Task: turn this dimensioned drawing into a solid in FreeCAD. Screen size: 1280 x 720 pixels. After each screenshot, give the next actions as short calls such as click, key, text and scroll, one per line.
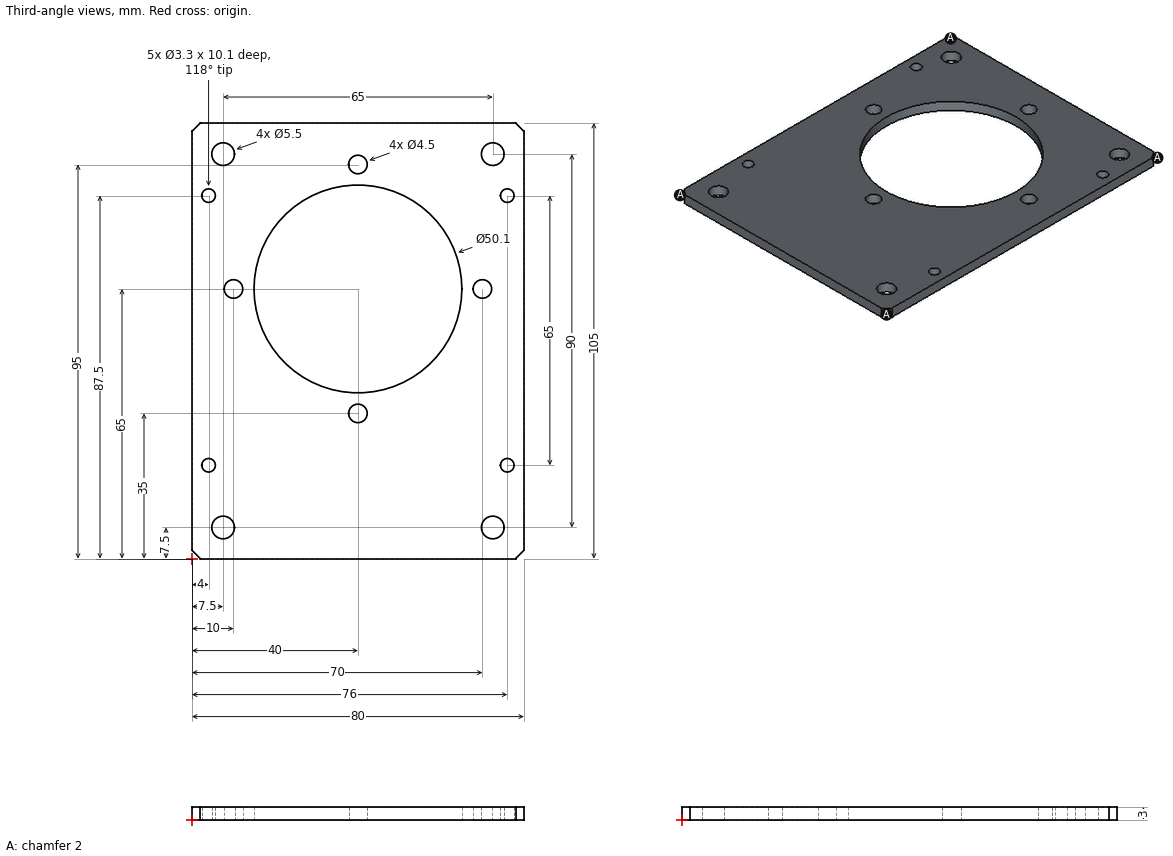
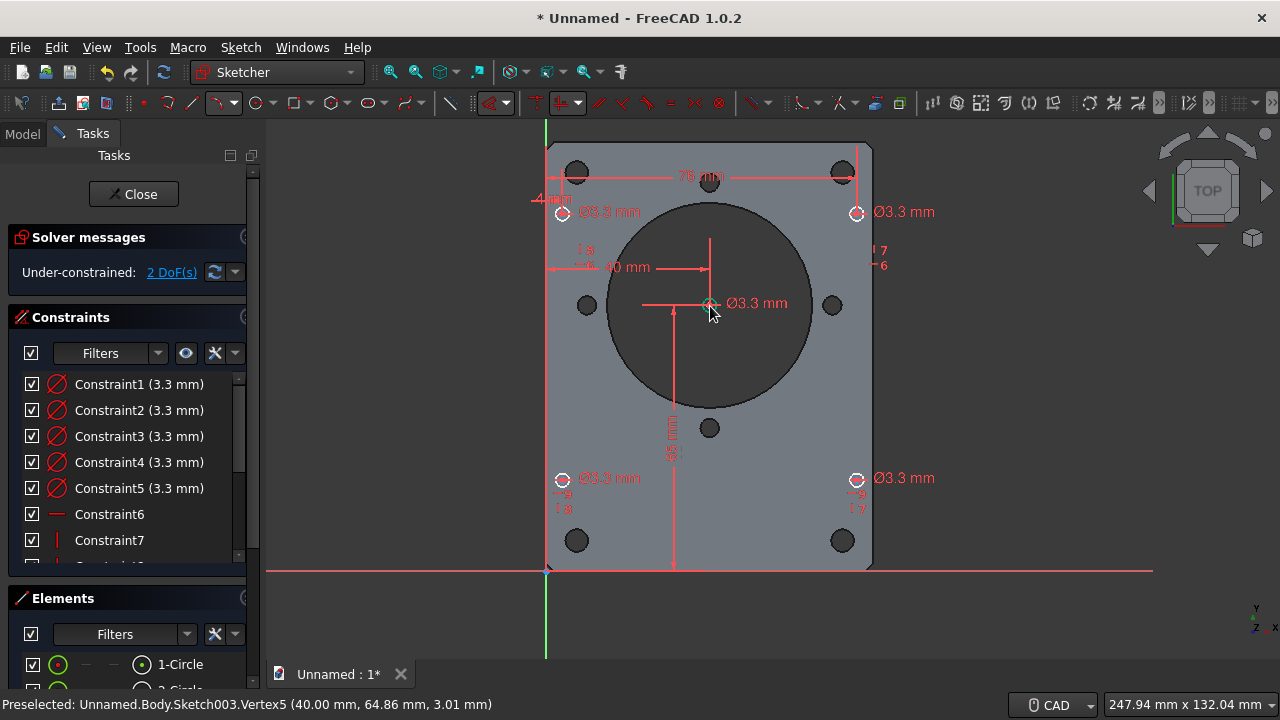
click(857, 214)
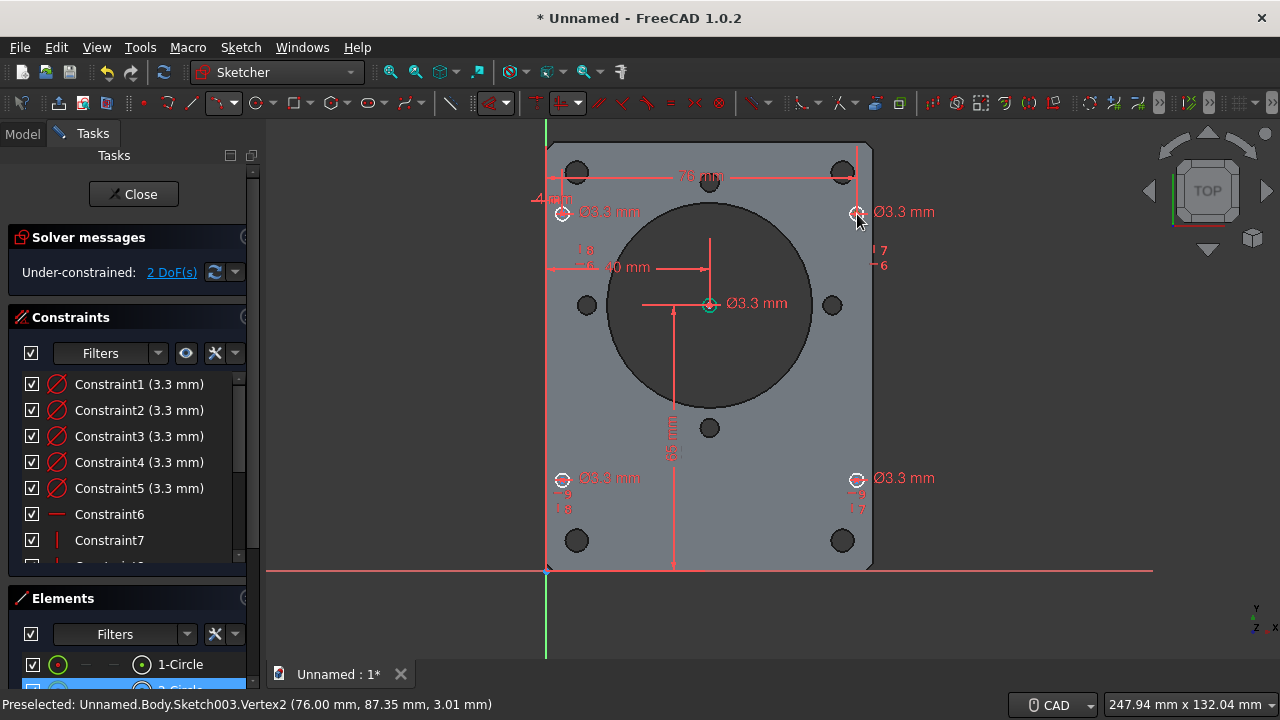
click(857, 480)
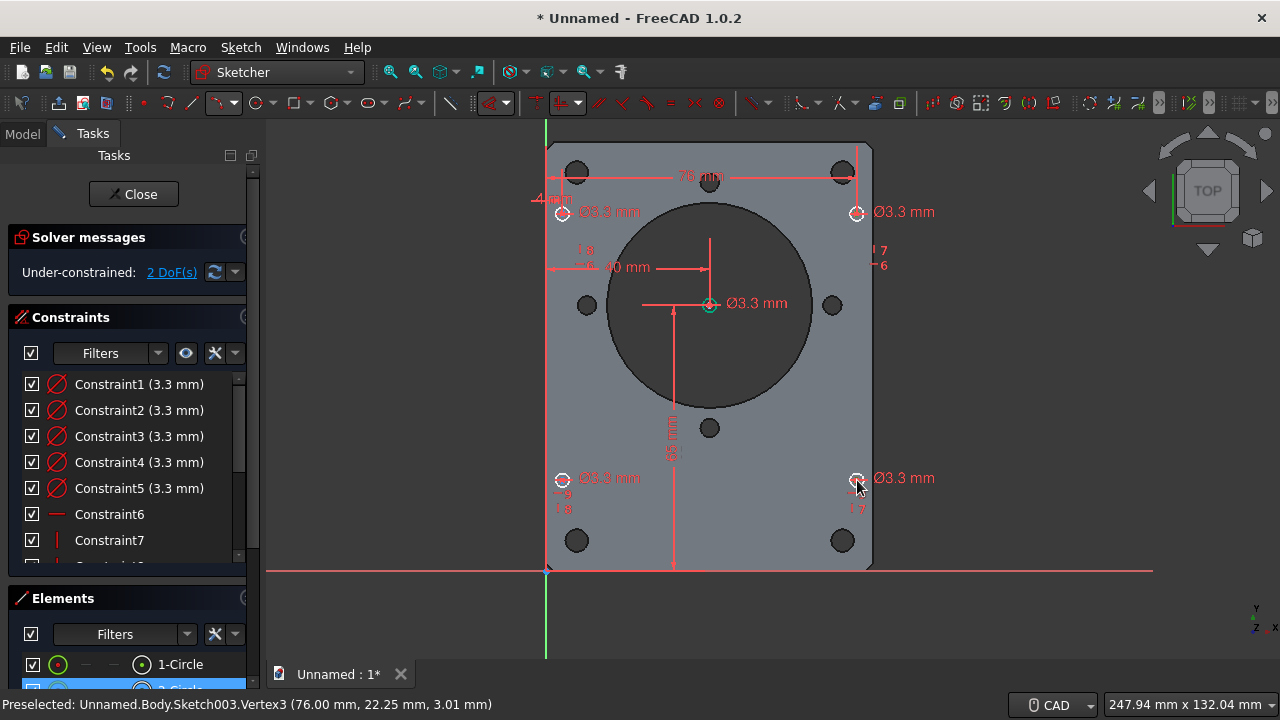
key(i)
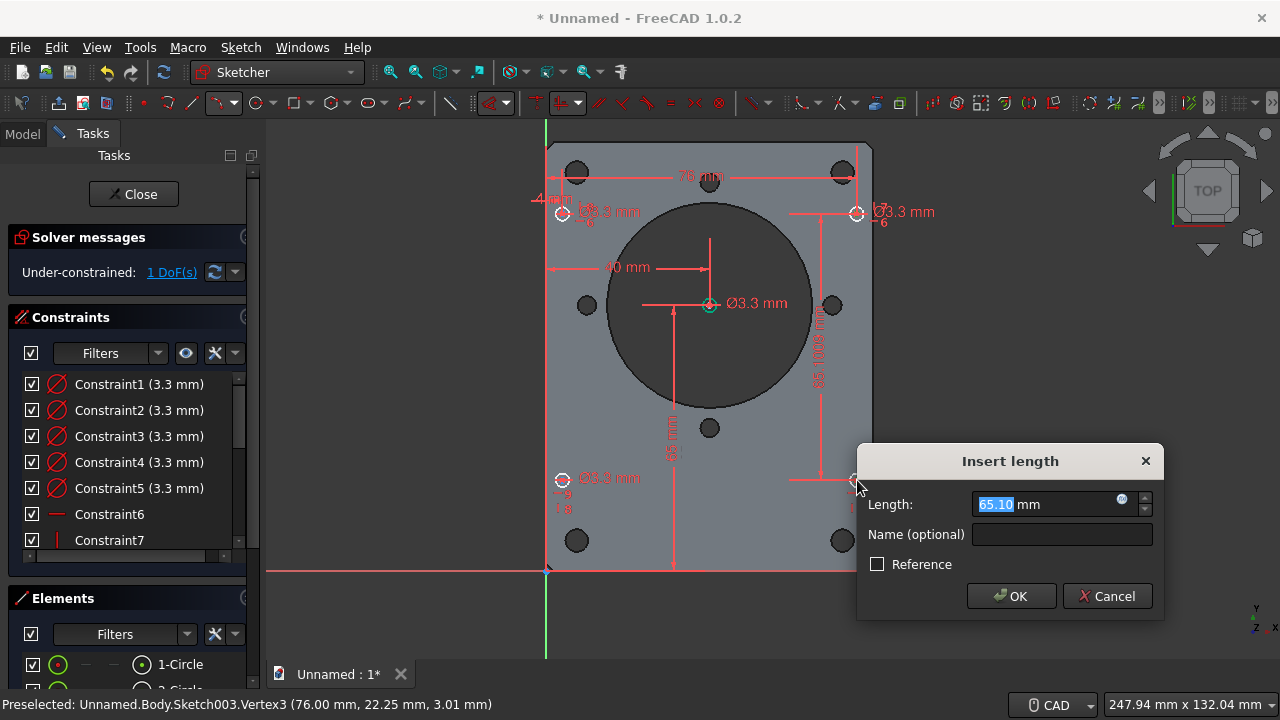
text(65)
key(Return)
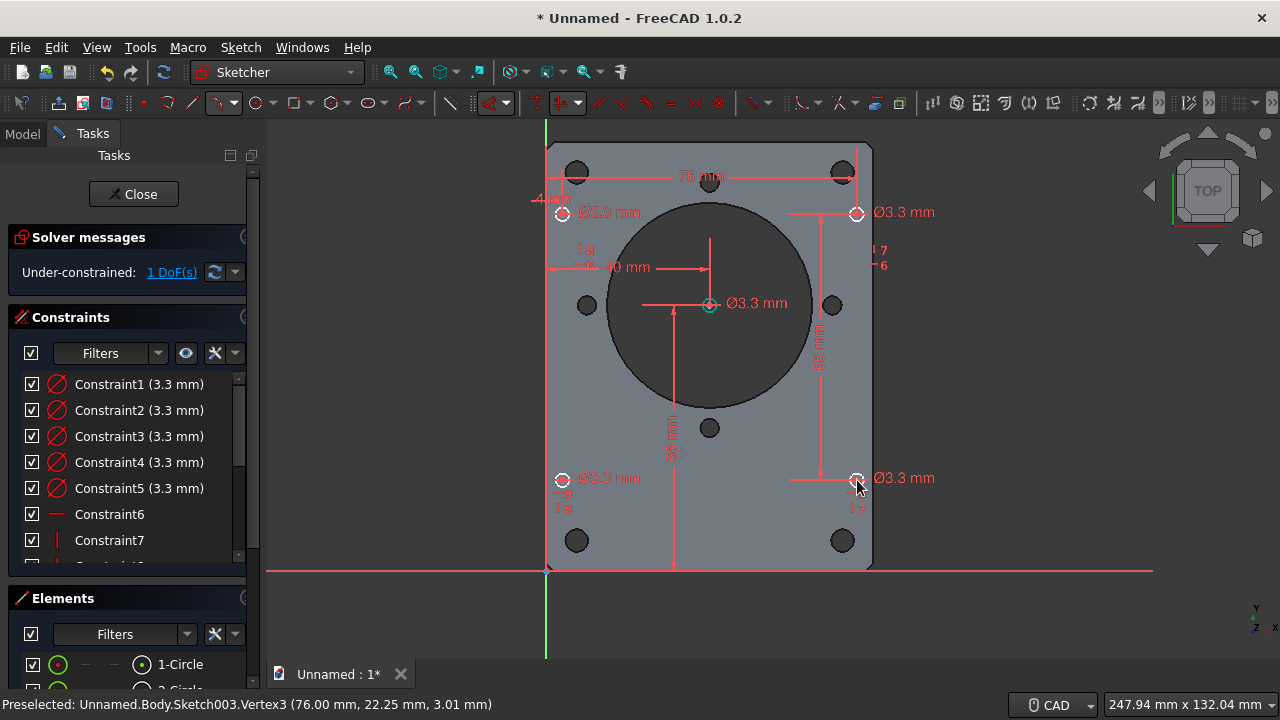
click(562, 214)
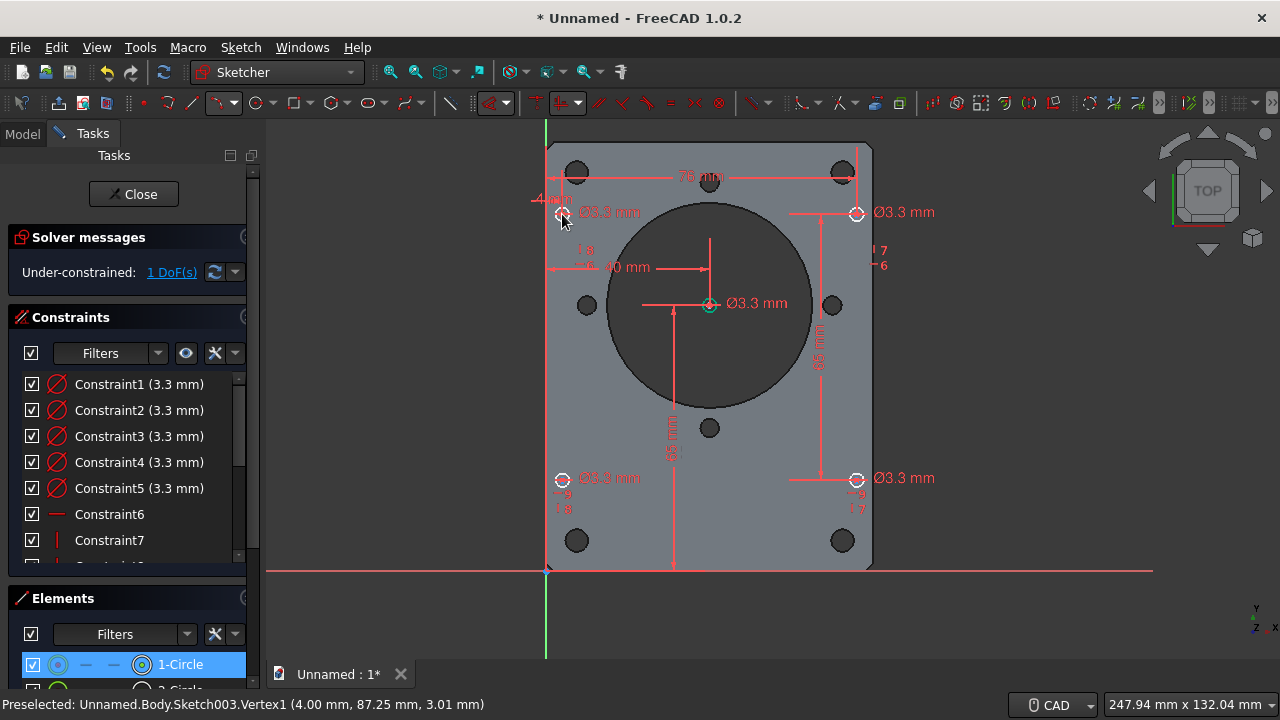
key(i)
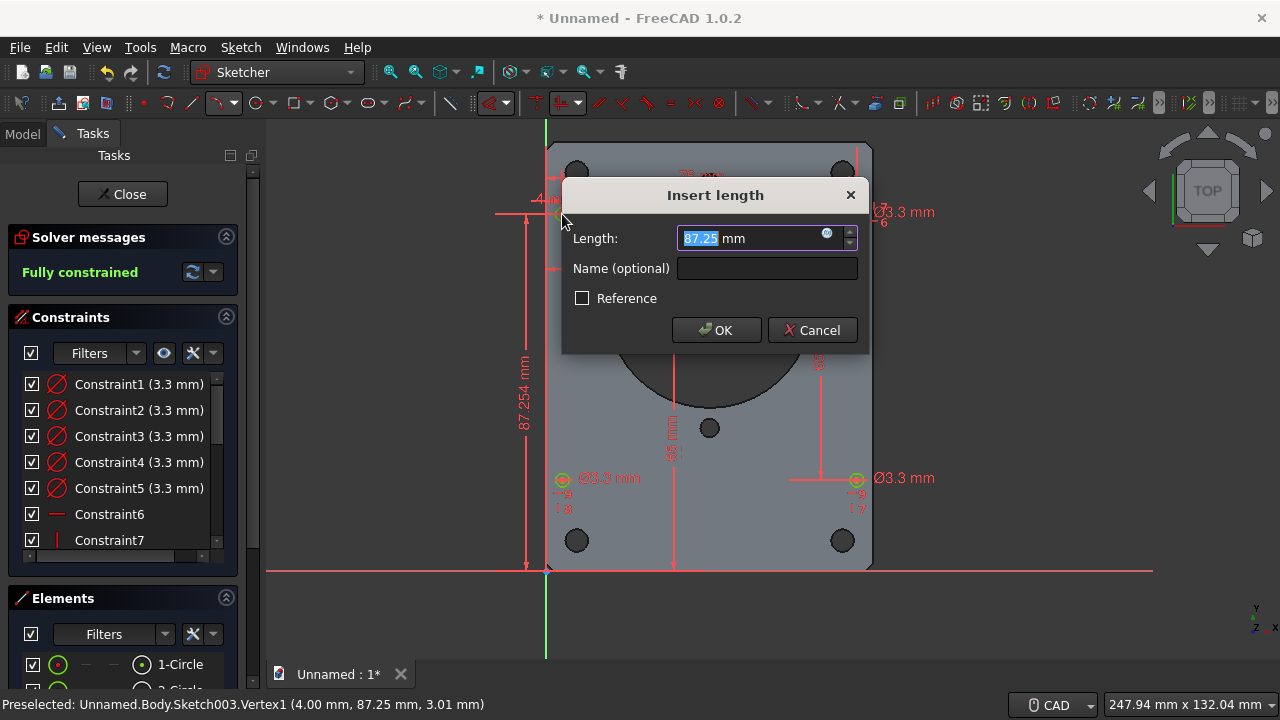
text(87.5)
key(Return)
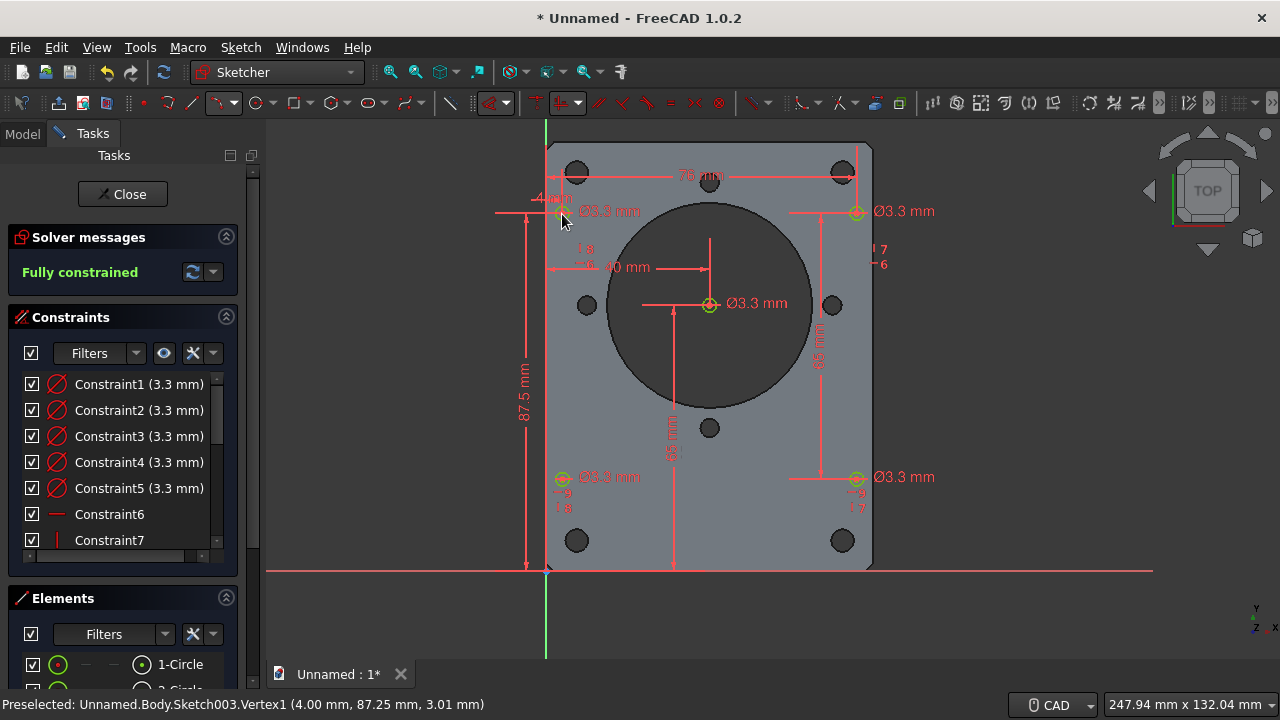
click(123, 194)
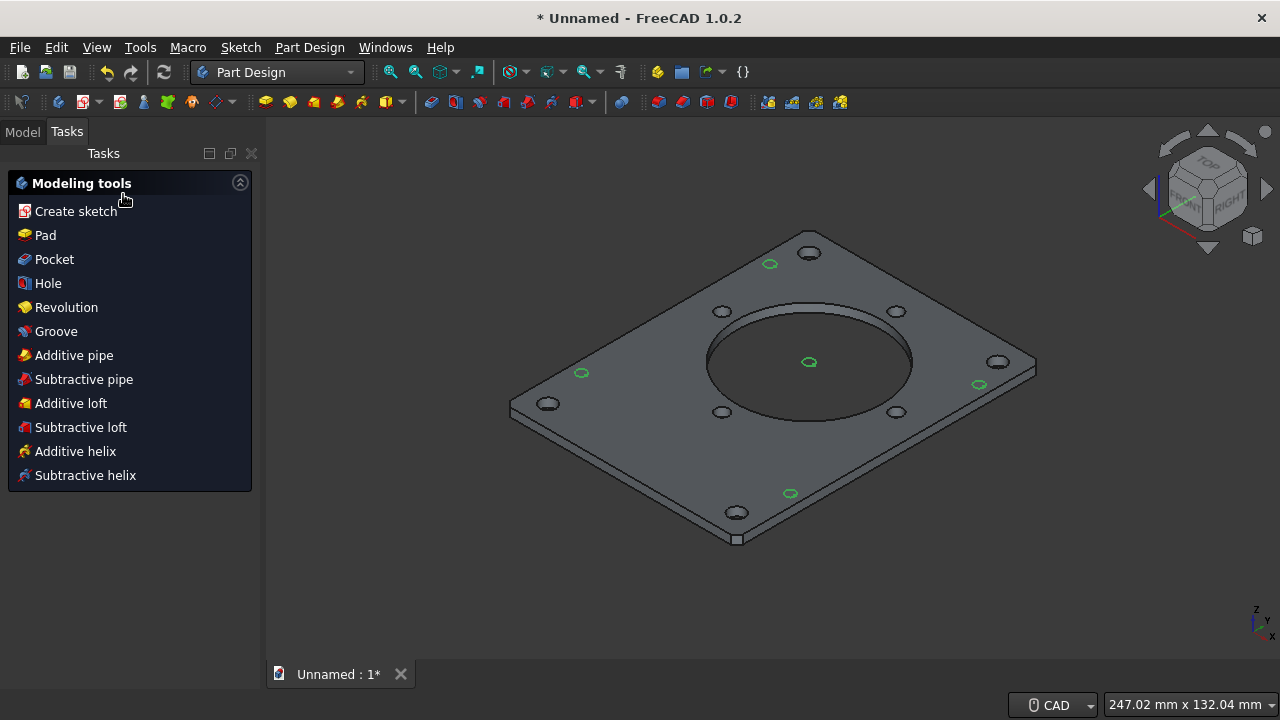
click(456, 102)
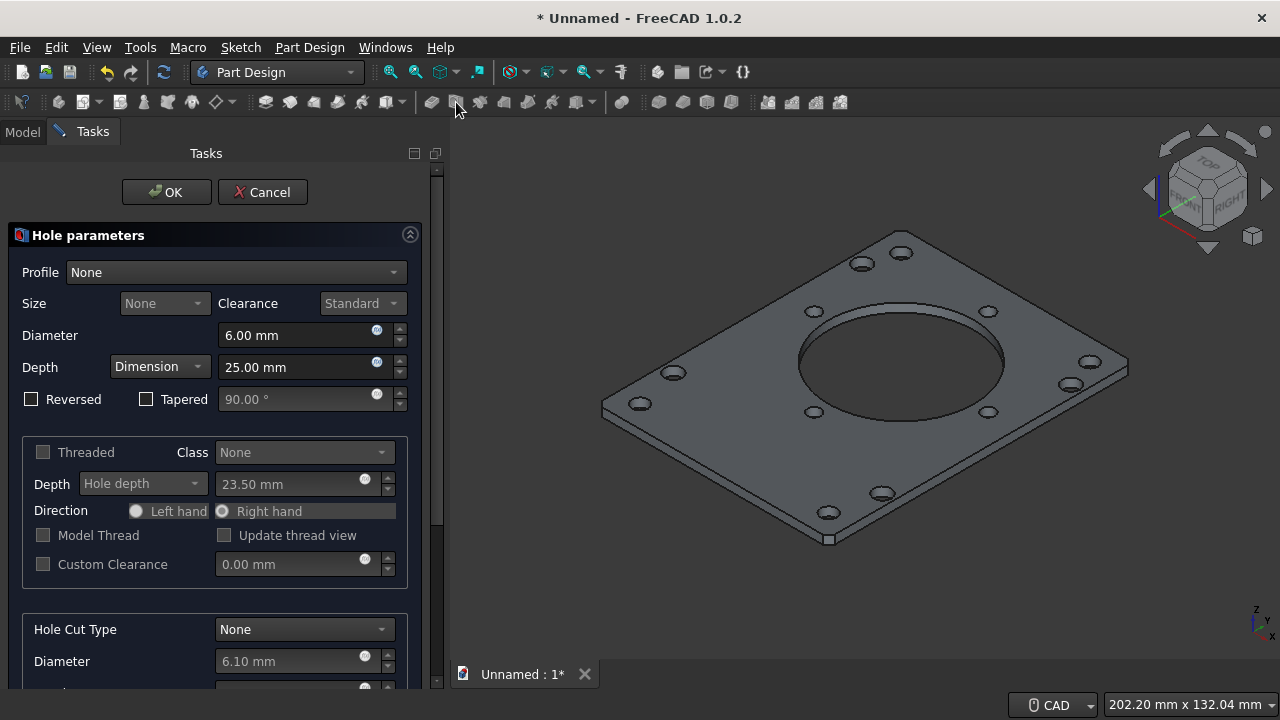
triple_click(305, 335)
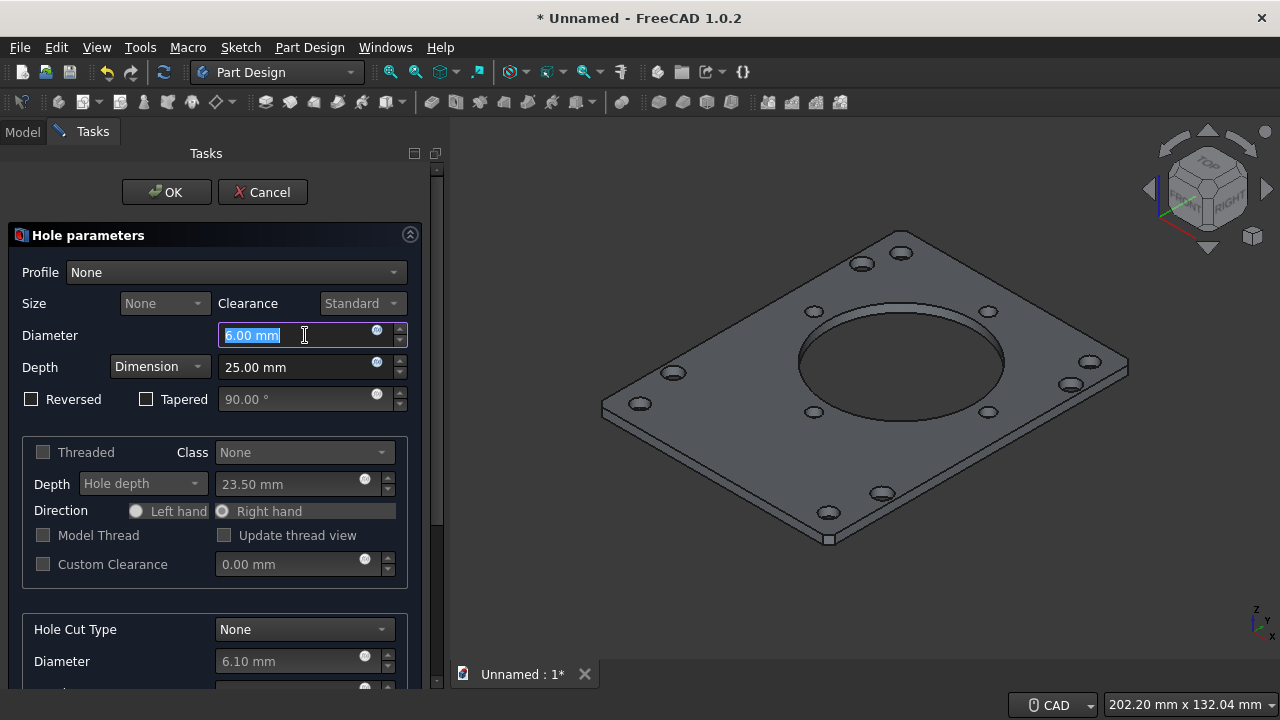
text(3.3)
key(Tab)